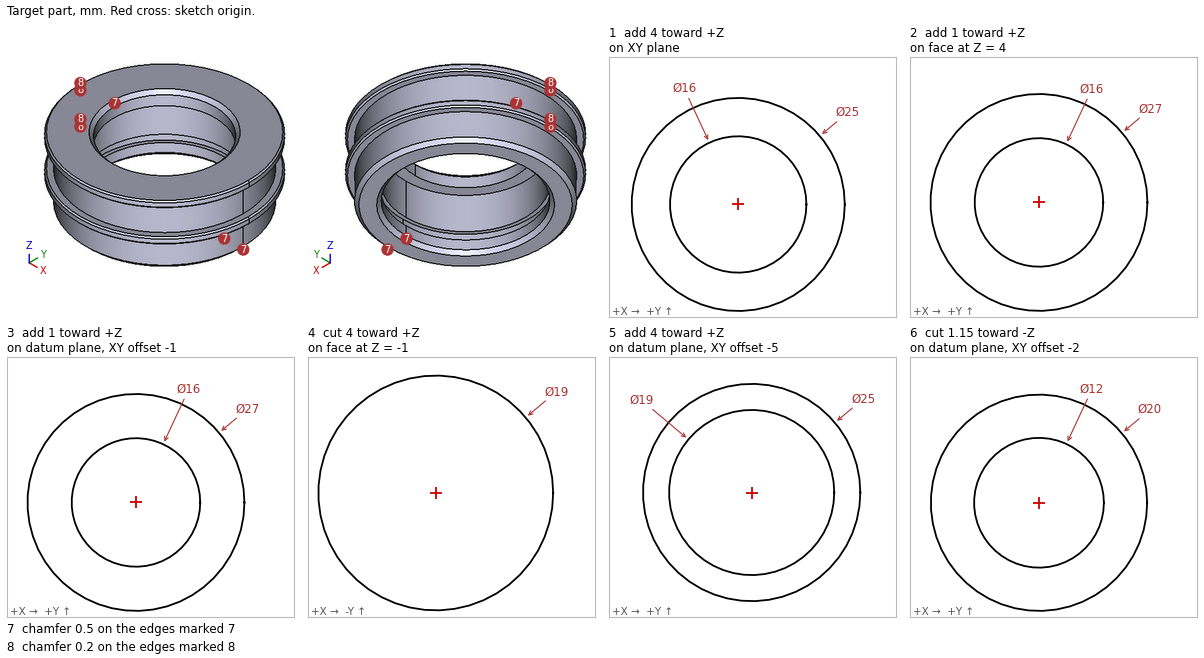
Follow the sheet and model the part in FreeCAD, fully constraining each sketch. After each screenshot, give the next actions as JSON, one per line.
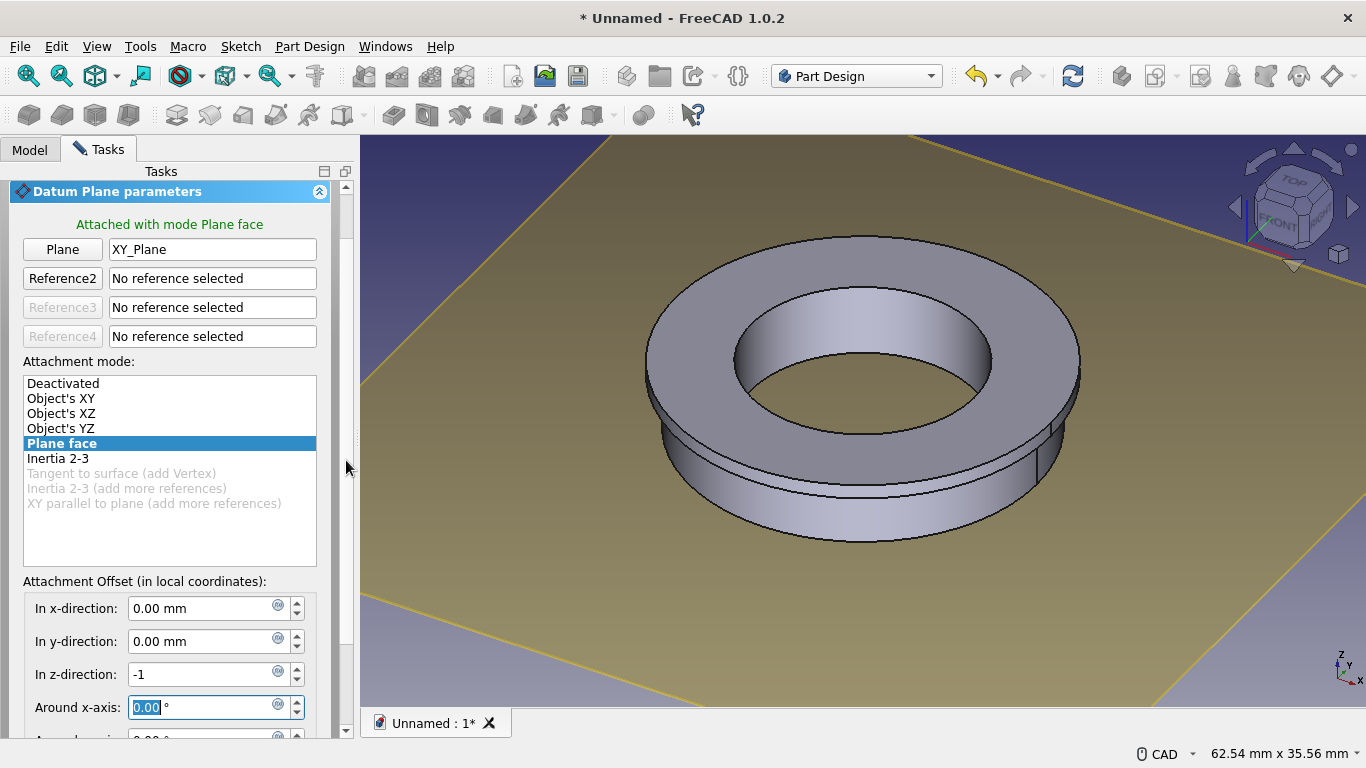
{"action": "left_click", "coordinate": [127, 210]}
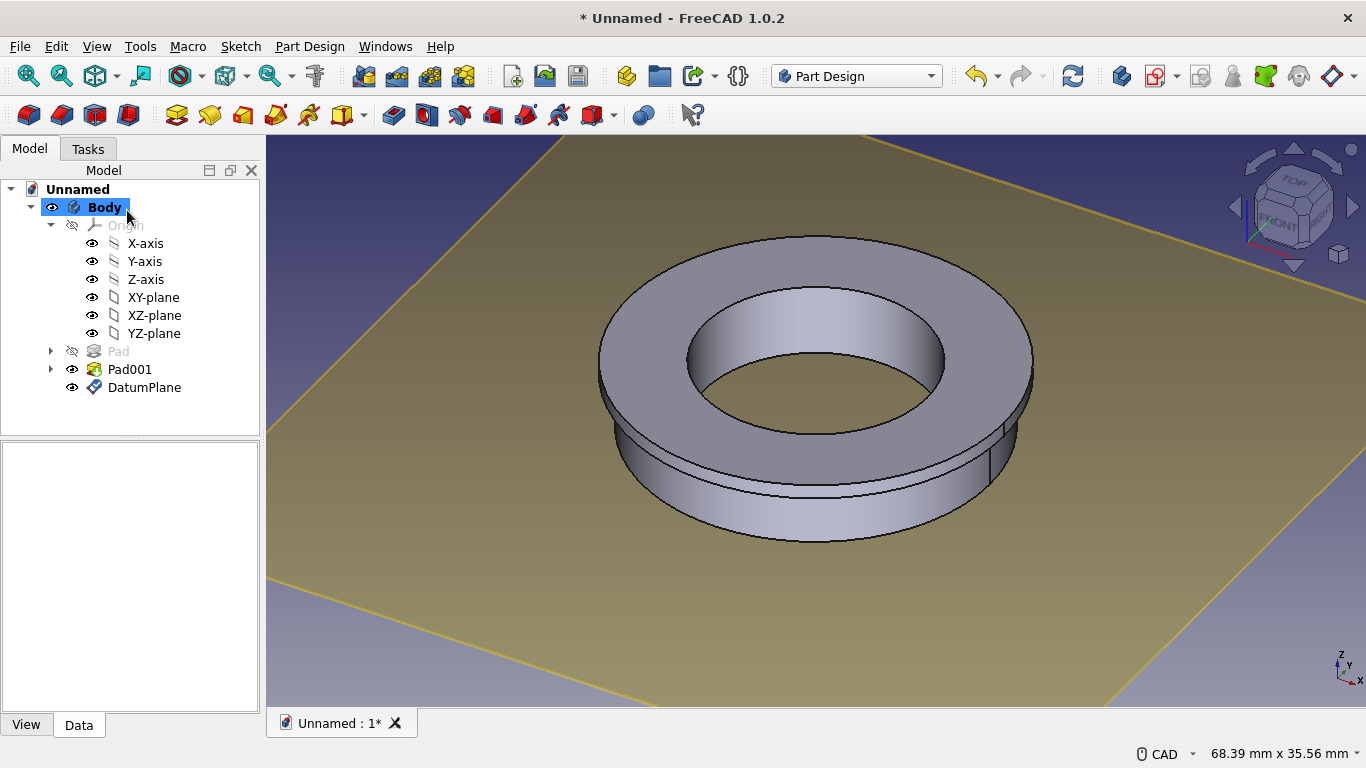
{"action": "left_click", "coordinate": [117, 387]}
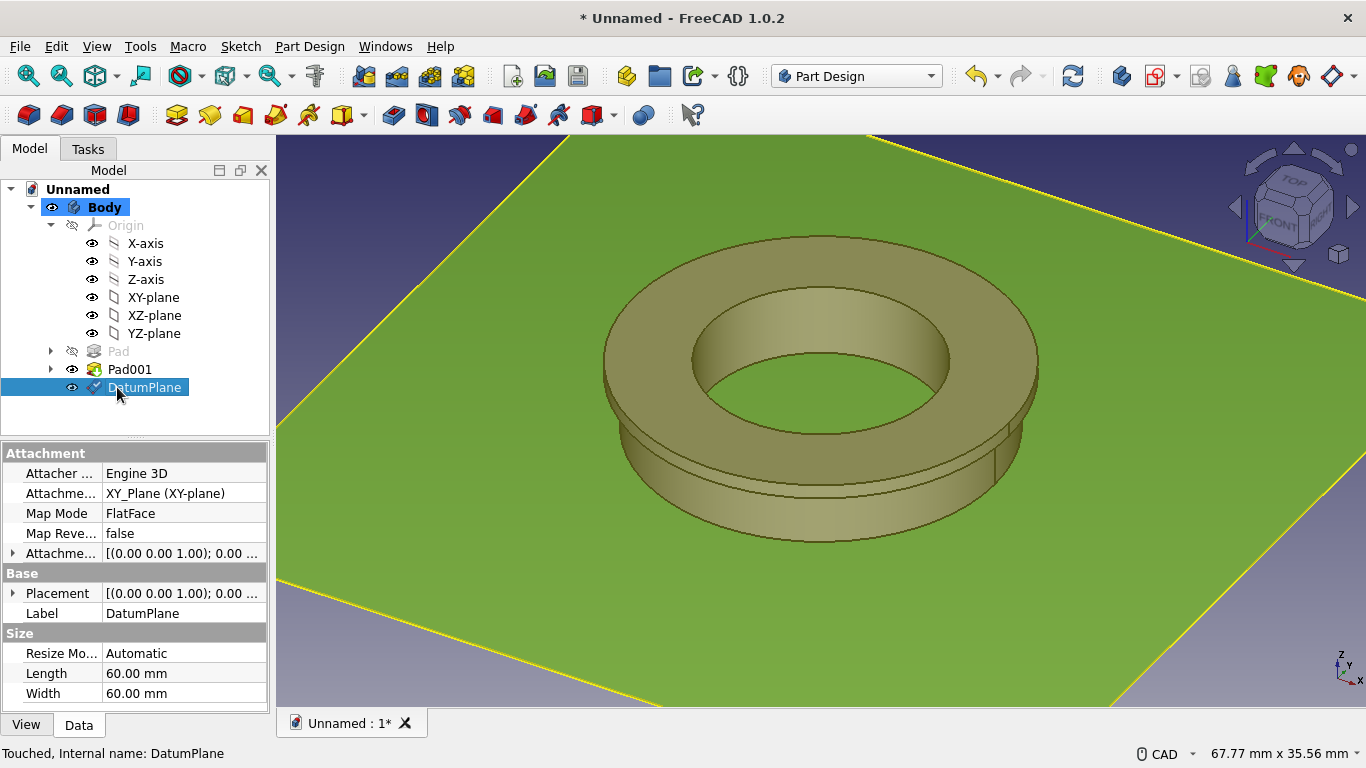
{"action": "left_click", "coordinate": [1154, 76]}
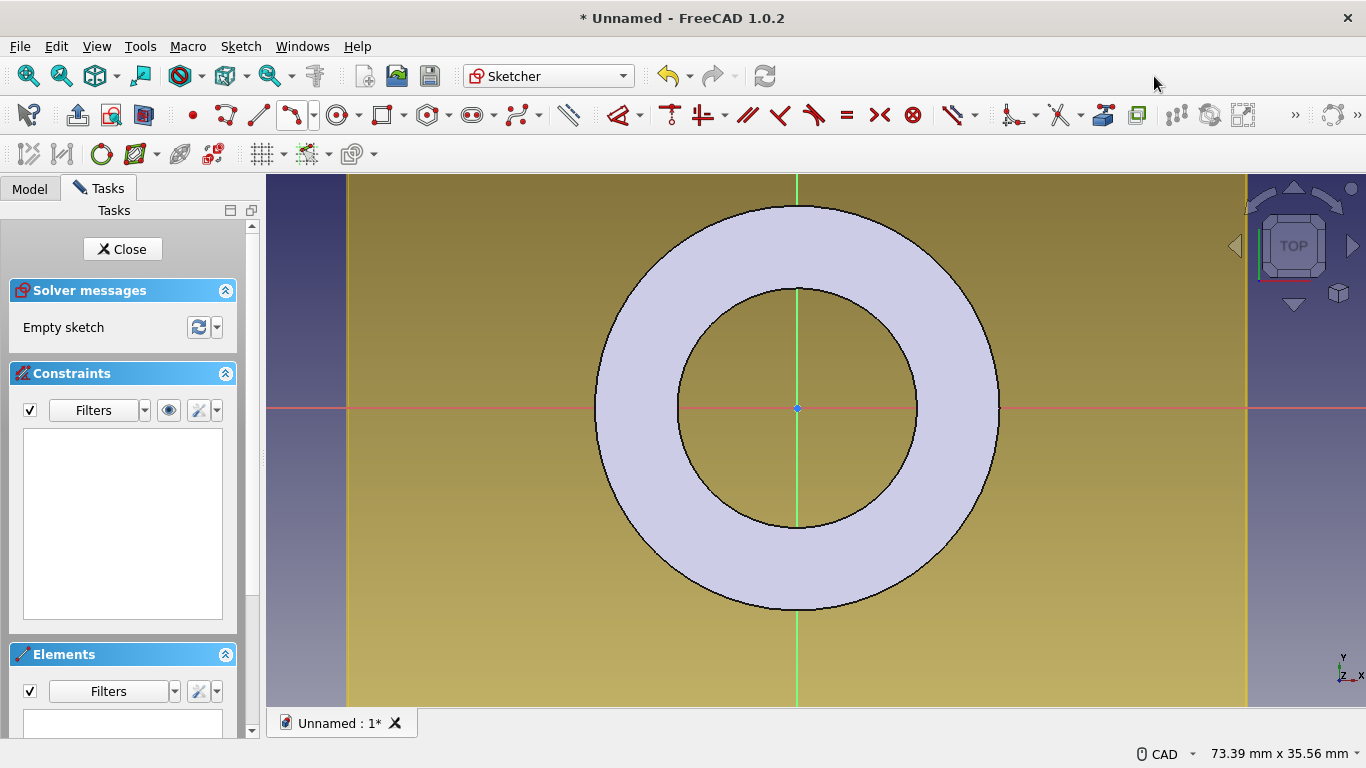
{"action": "left_click", "coordinate": [144, 116]}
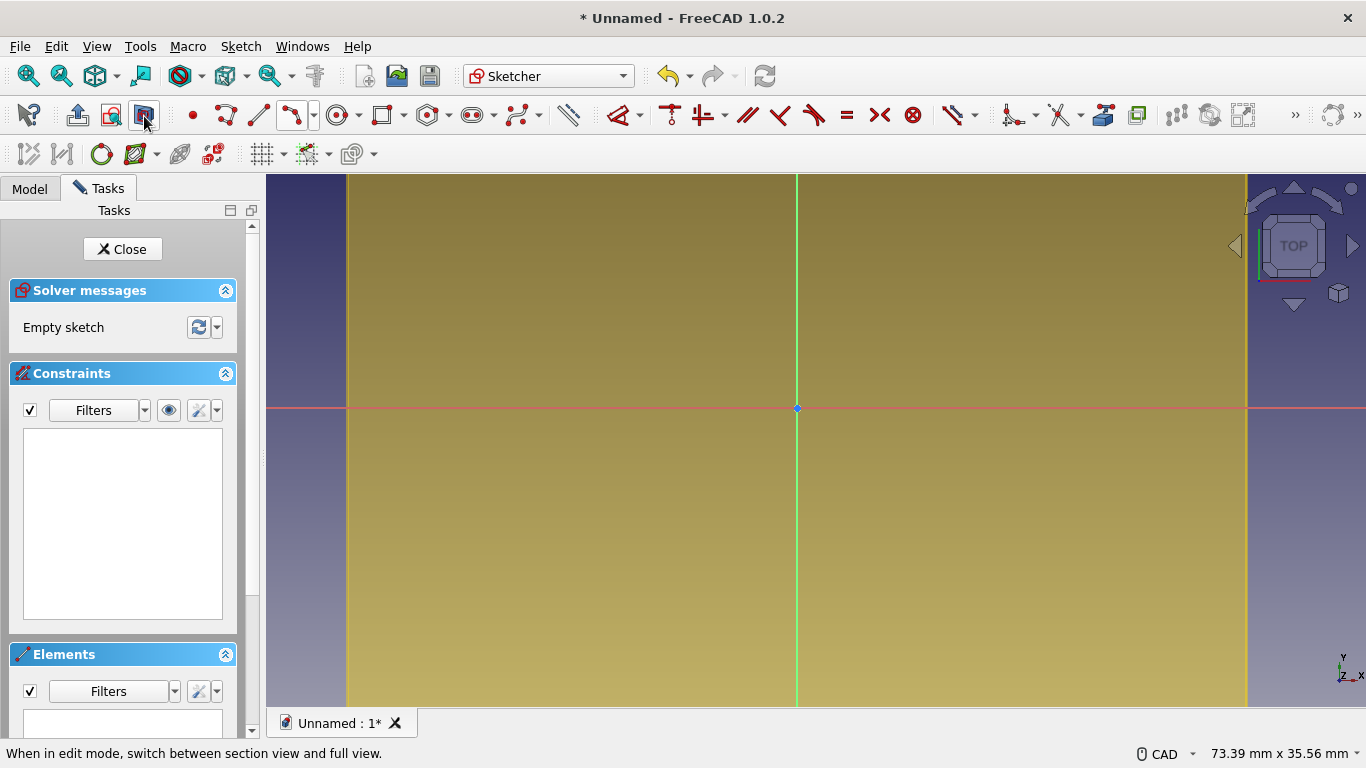
{"action": "scroll", "coordinate": [523, 587], "scroll_direction": "down", "scroll_amount": 1}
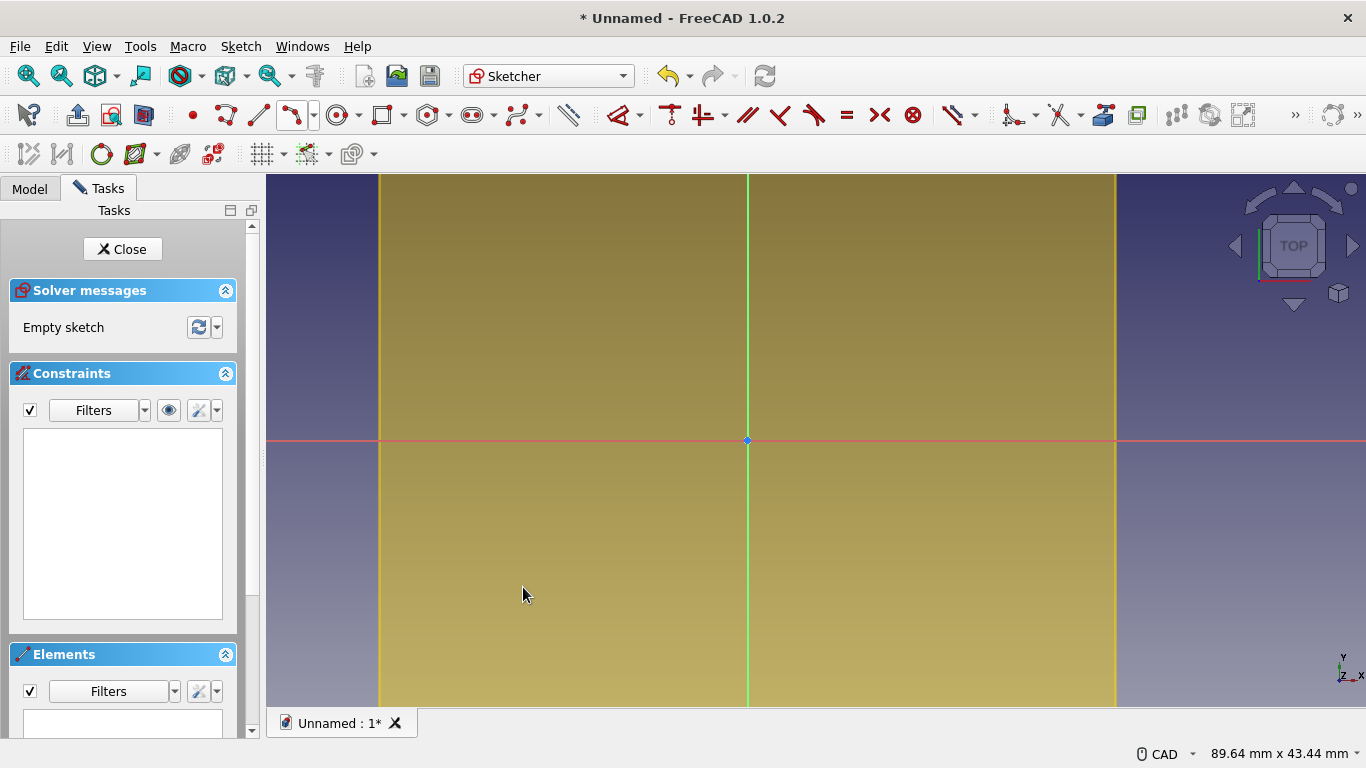
{"action": "left_click", "coordinate": [336, 116]}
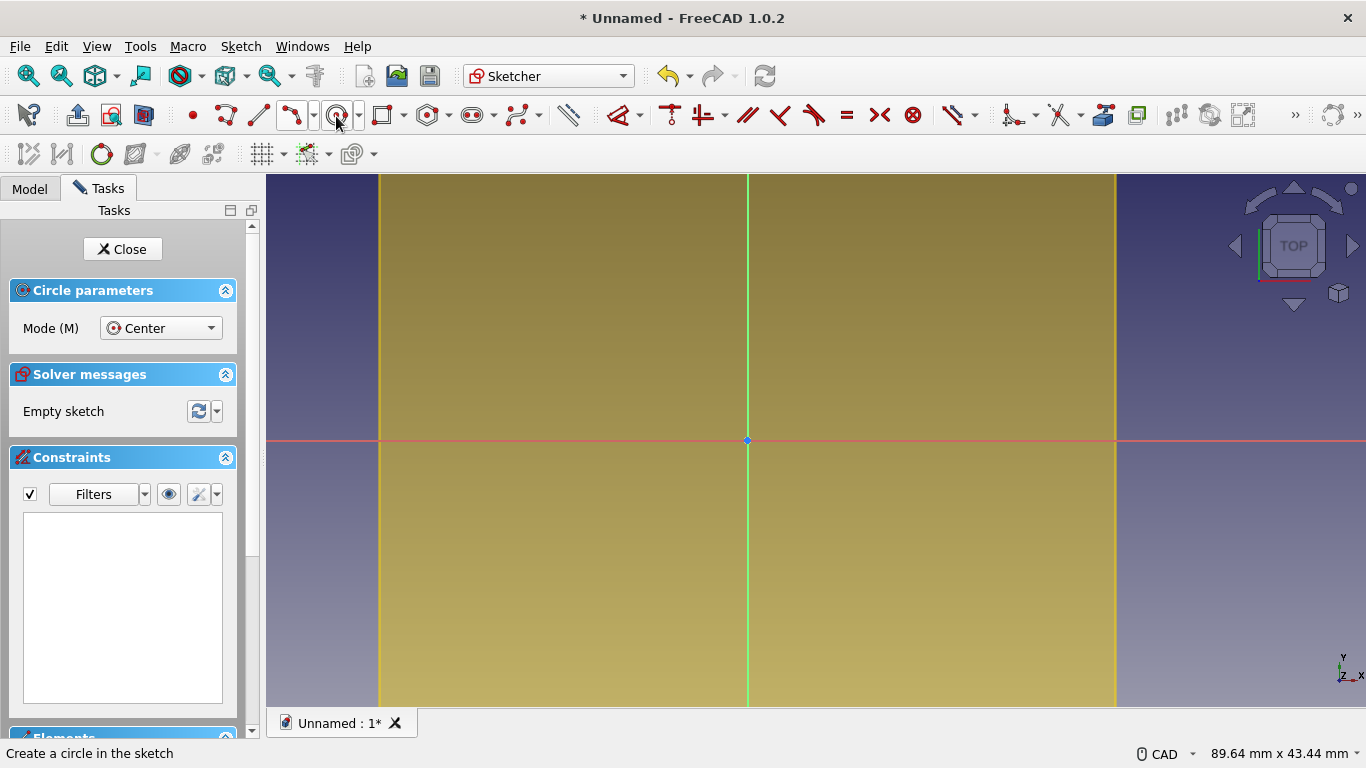
{"action": "left_click", "coordinate": [748, 441]}
{"action": "left_click", "coordinate": [865, 324]}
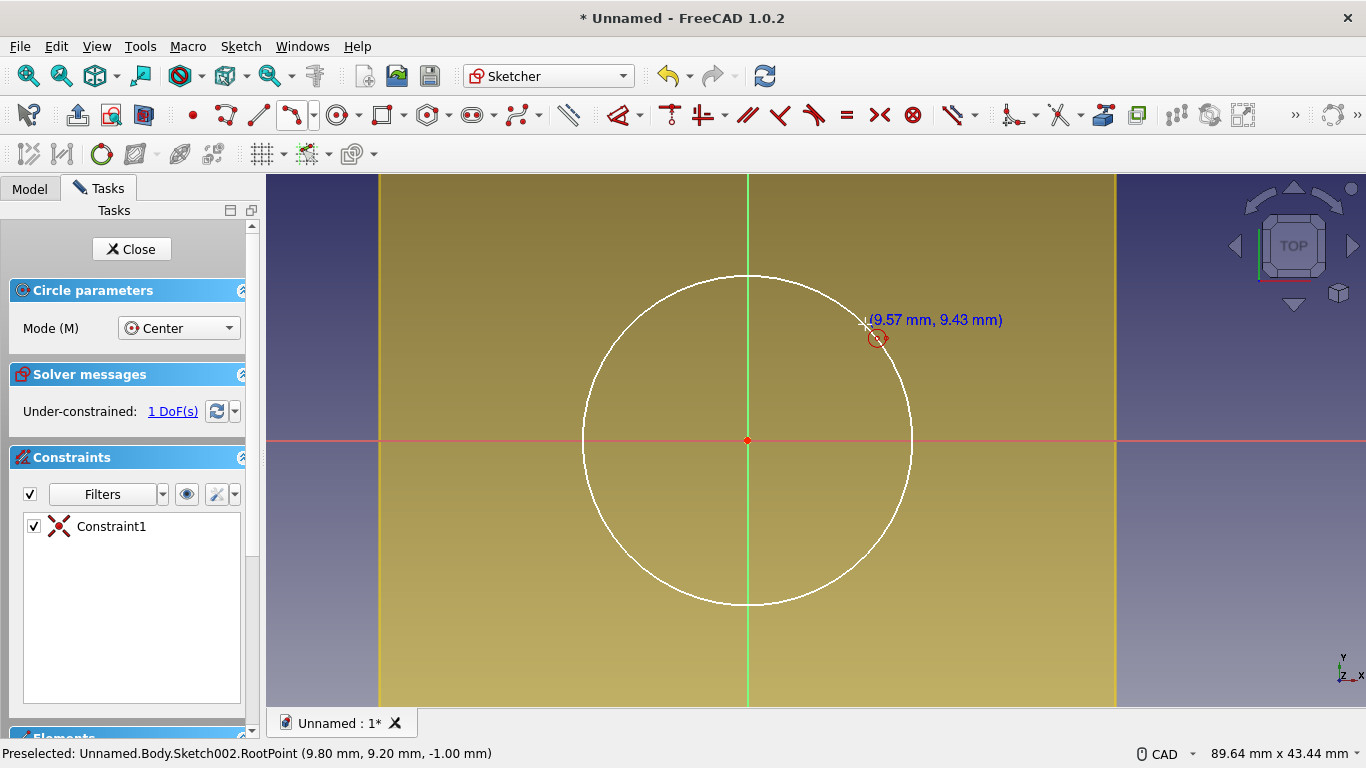
{"action": "left_click", "coordinate": [748, 441]}
{"action": "left_click", "coordinate": [817, 371]}
{"action": "key", "text": "Escape"}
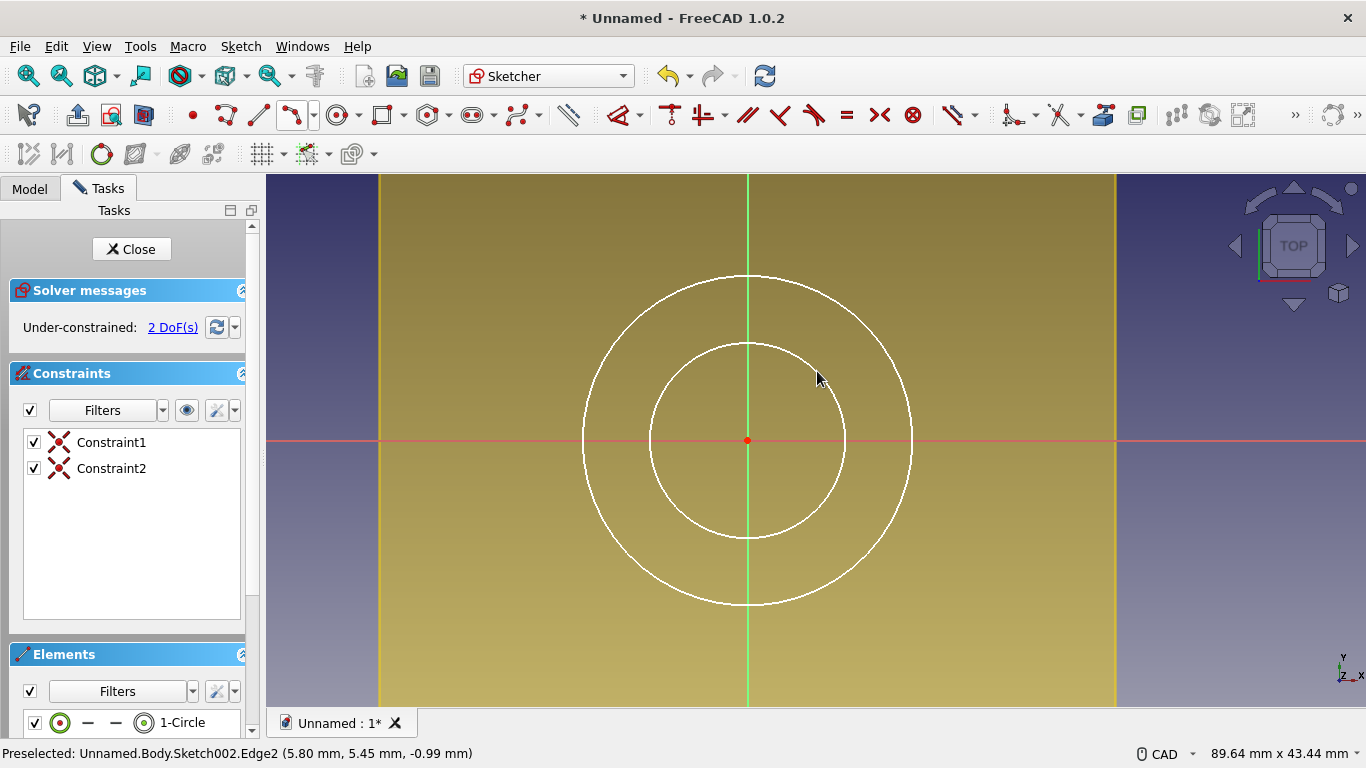
{"action": "left_click", "coordinate": [618, 116]}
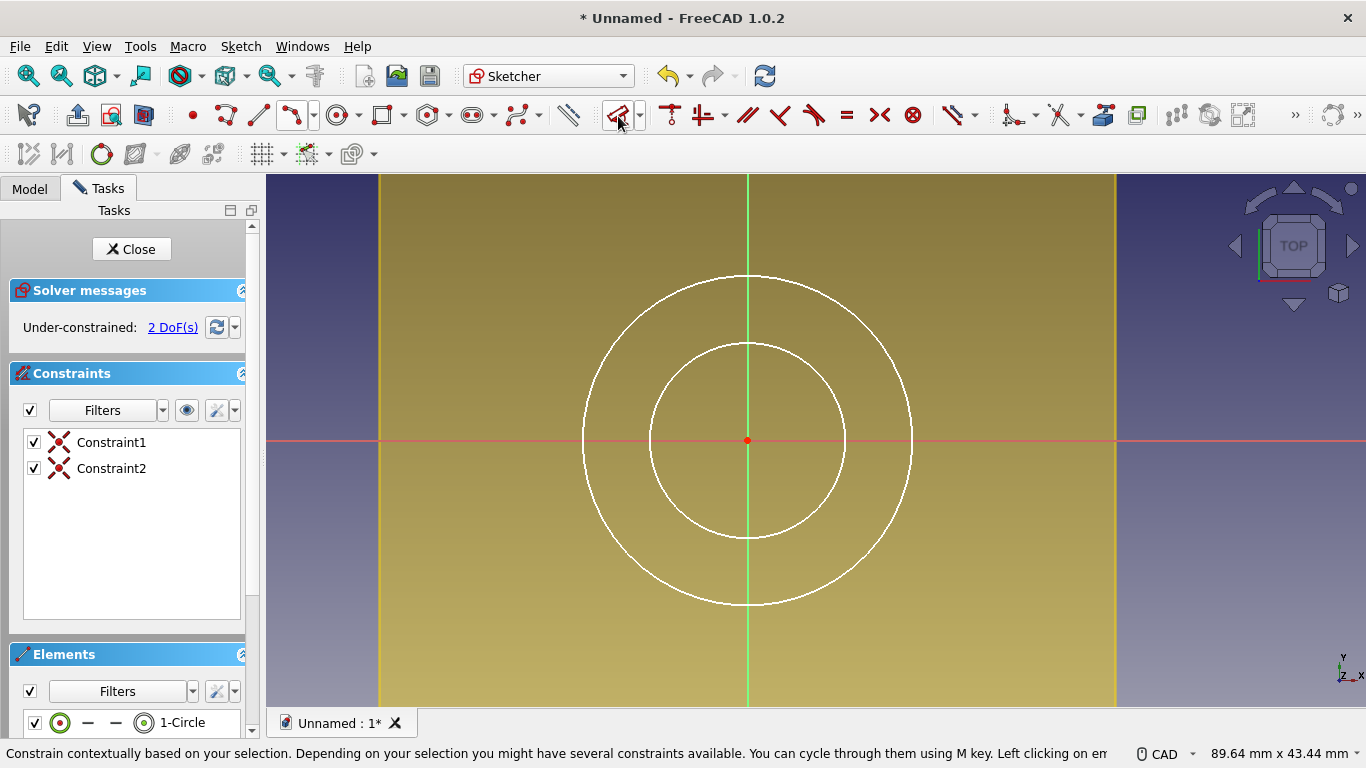
{"action": "left_click", "coordinate": [864, 324]}
{"action": "left_click", "coordinate": [887, 301]}